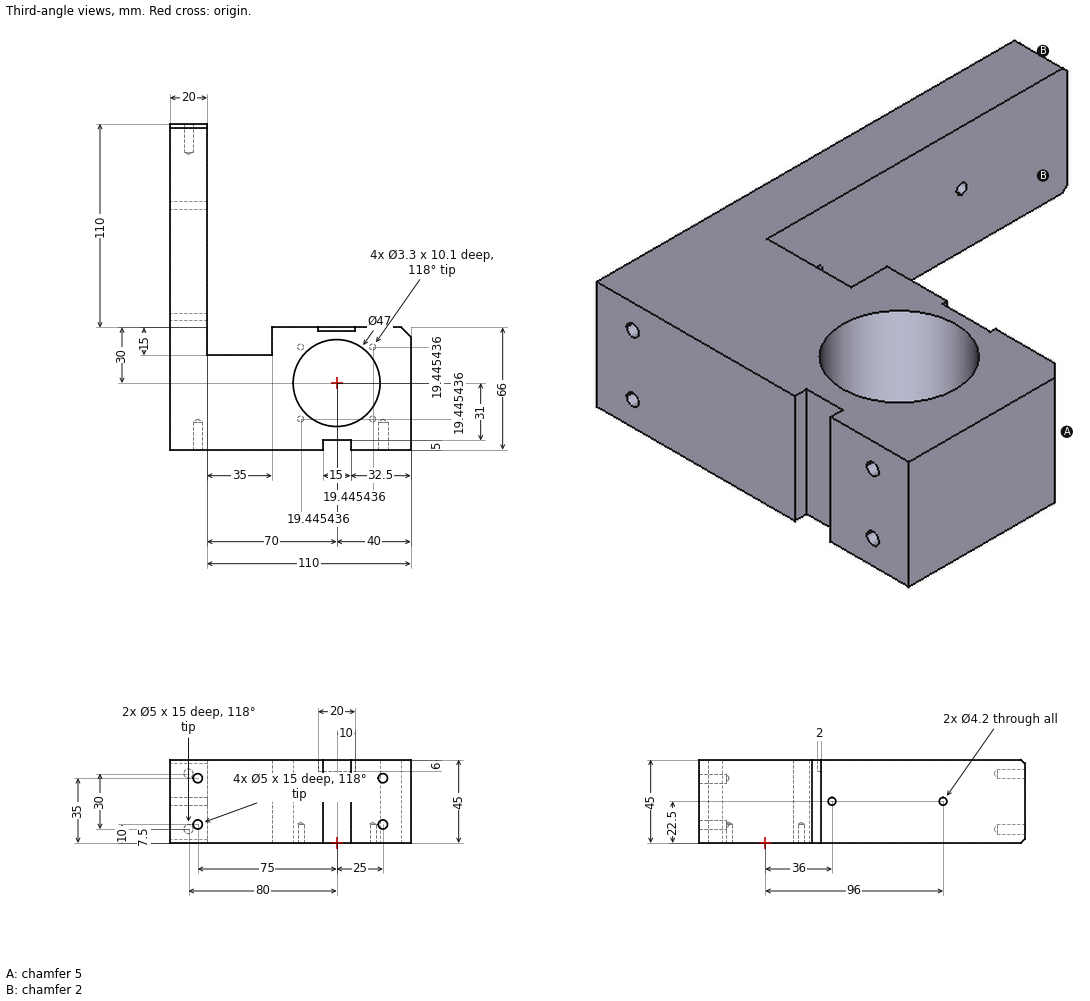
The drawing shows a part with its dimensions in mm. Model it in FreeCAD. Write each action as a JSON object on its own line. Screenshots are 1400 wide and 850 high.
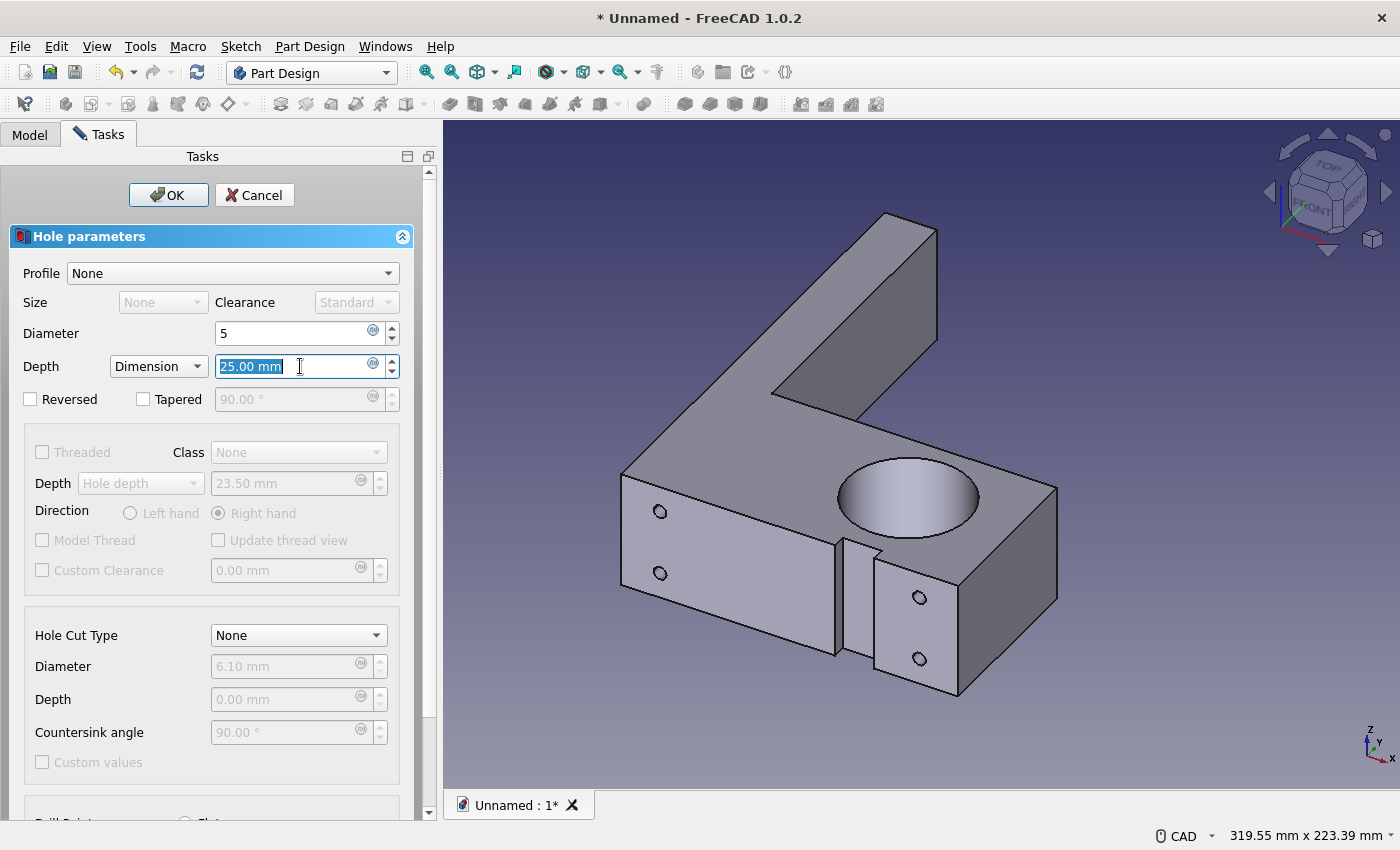
{"action": "type", "text": "15"}
{"action": "key", "text": "Tab"}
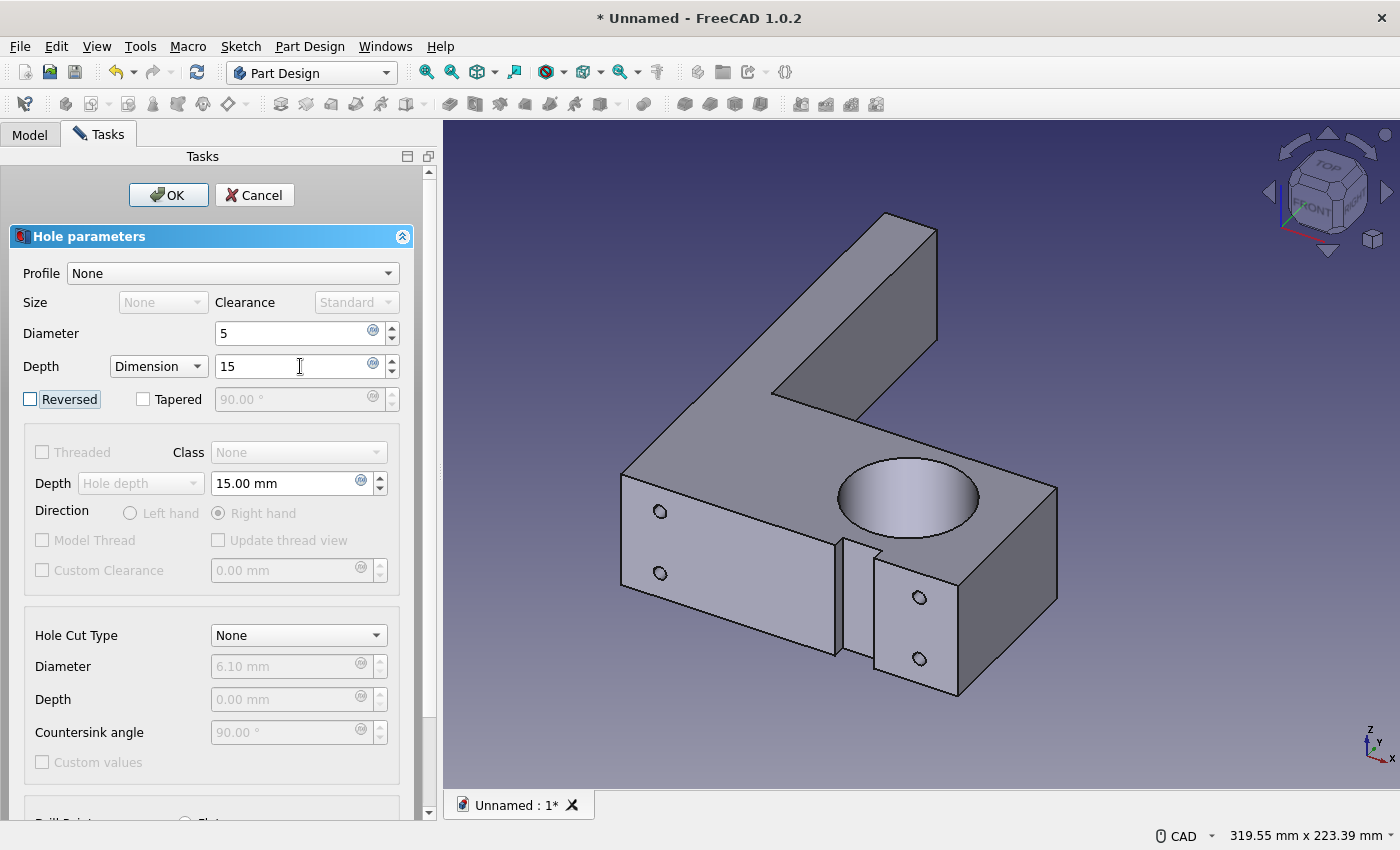
{"action": "left_click", "coordinate": [169, 195]}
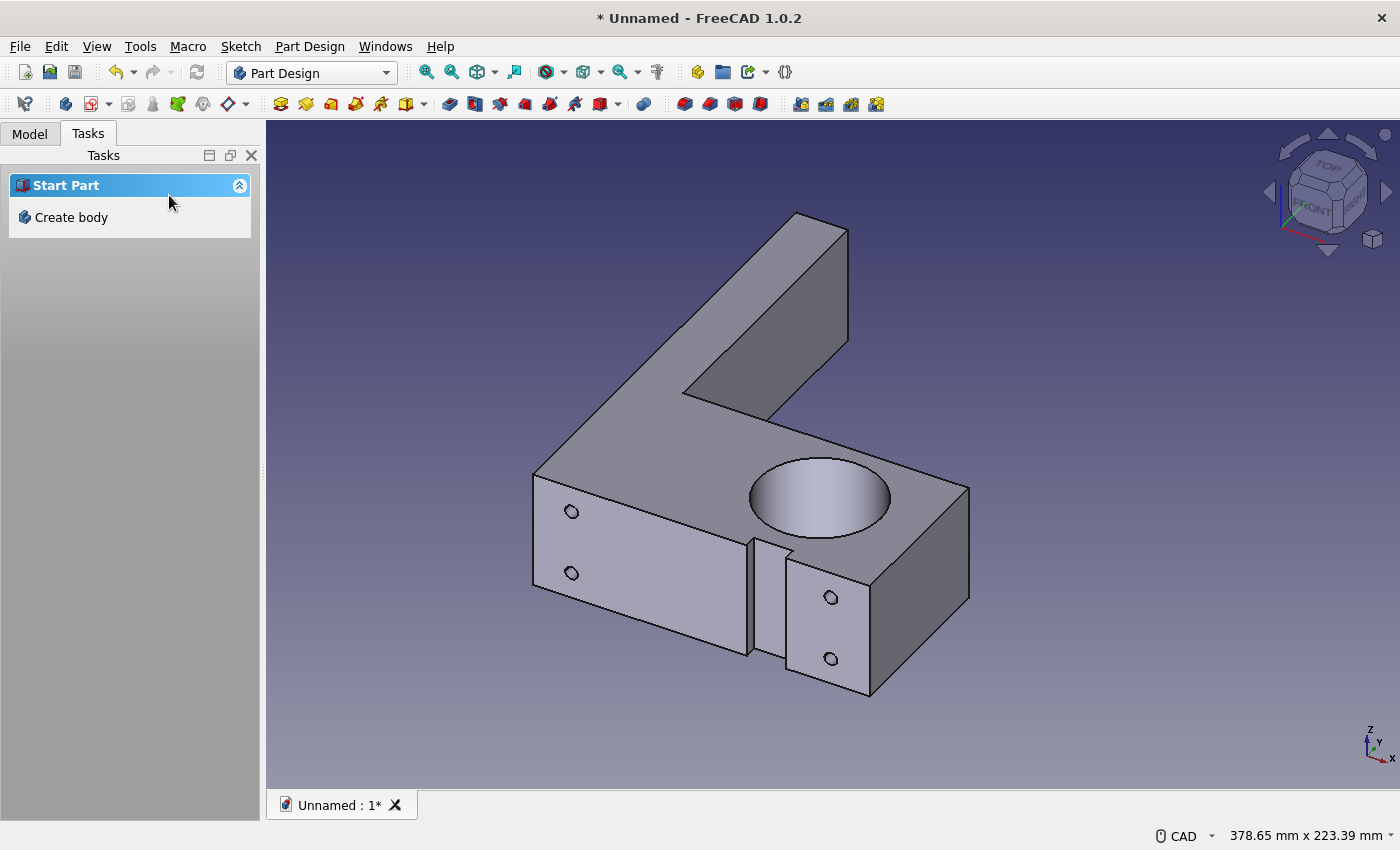
{"action": "left_click", "coordinate": [813, 319]}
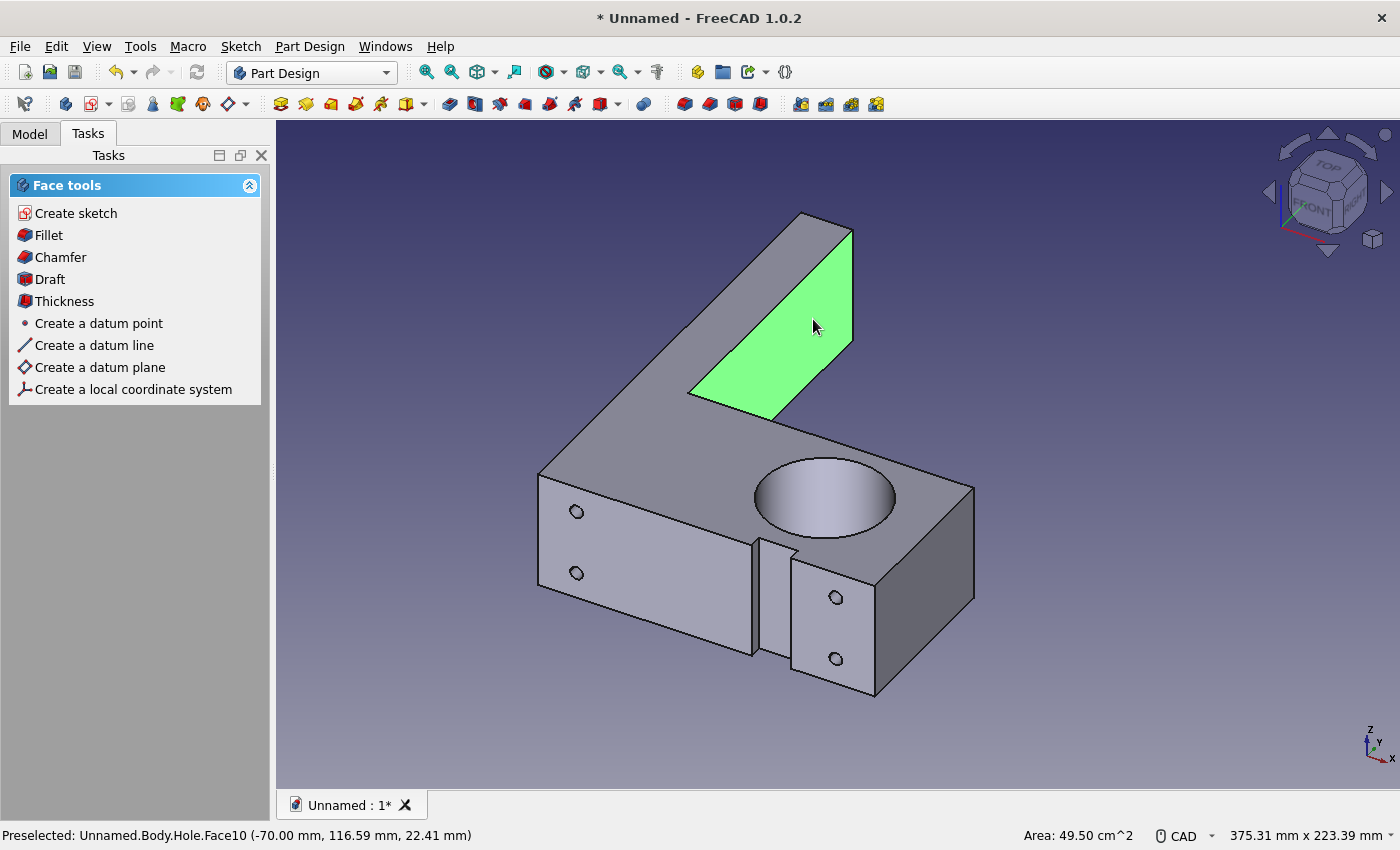
{"action": "left_click", "coordinate": [90, 104]}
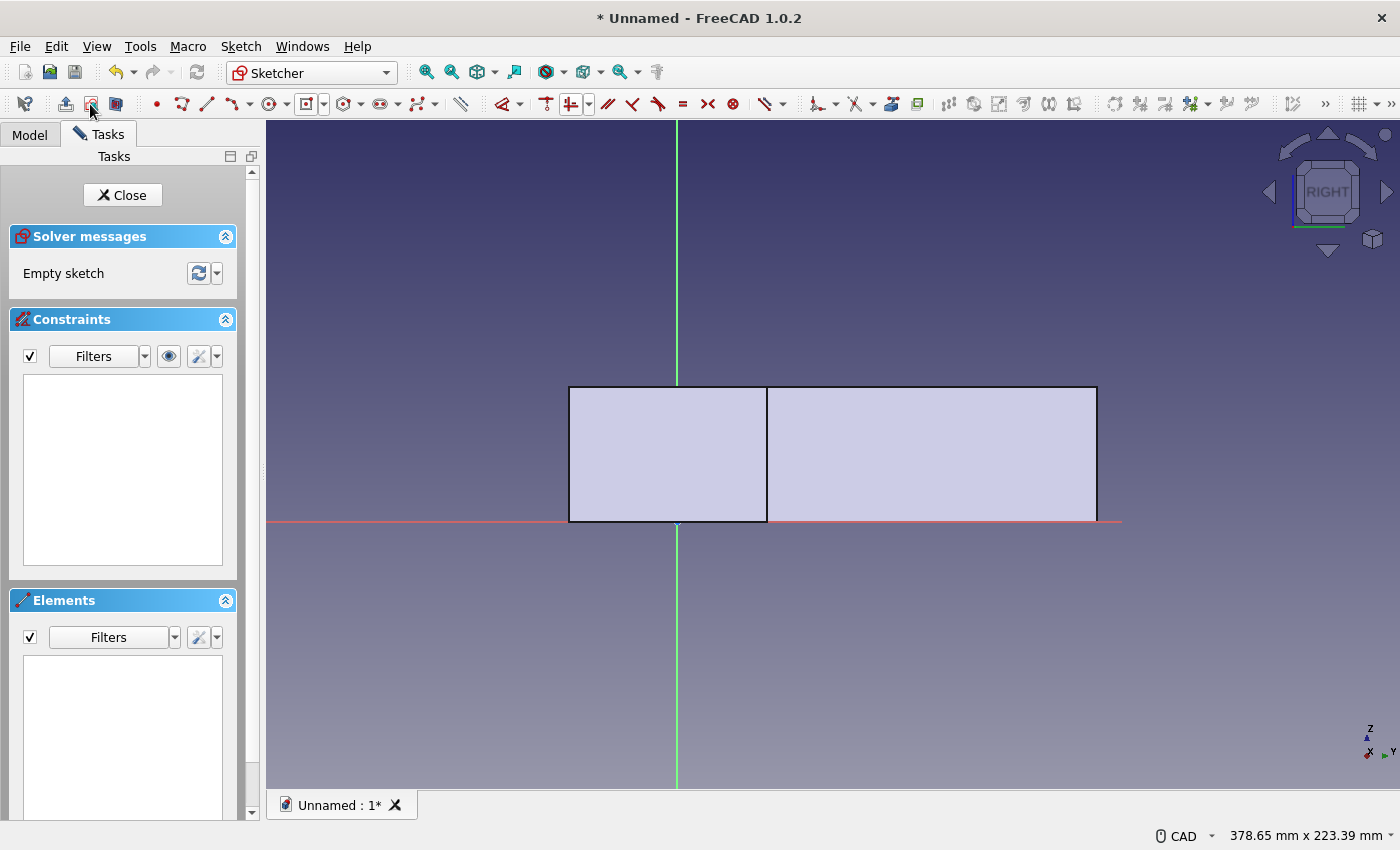
{"action": "left_click", "coordinate": [116, 104]}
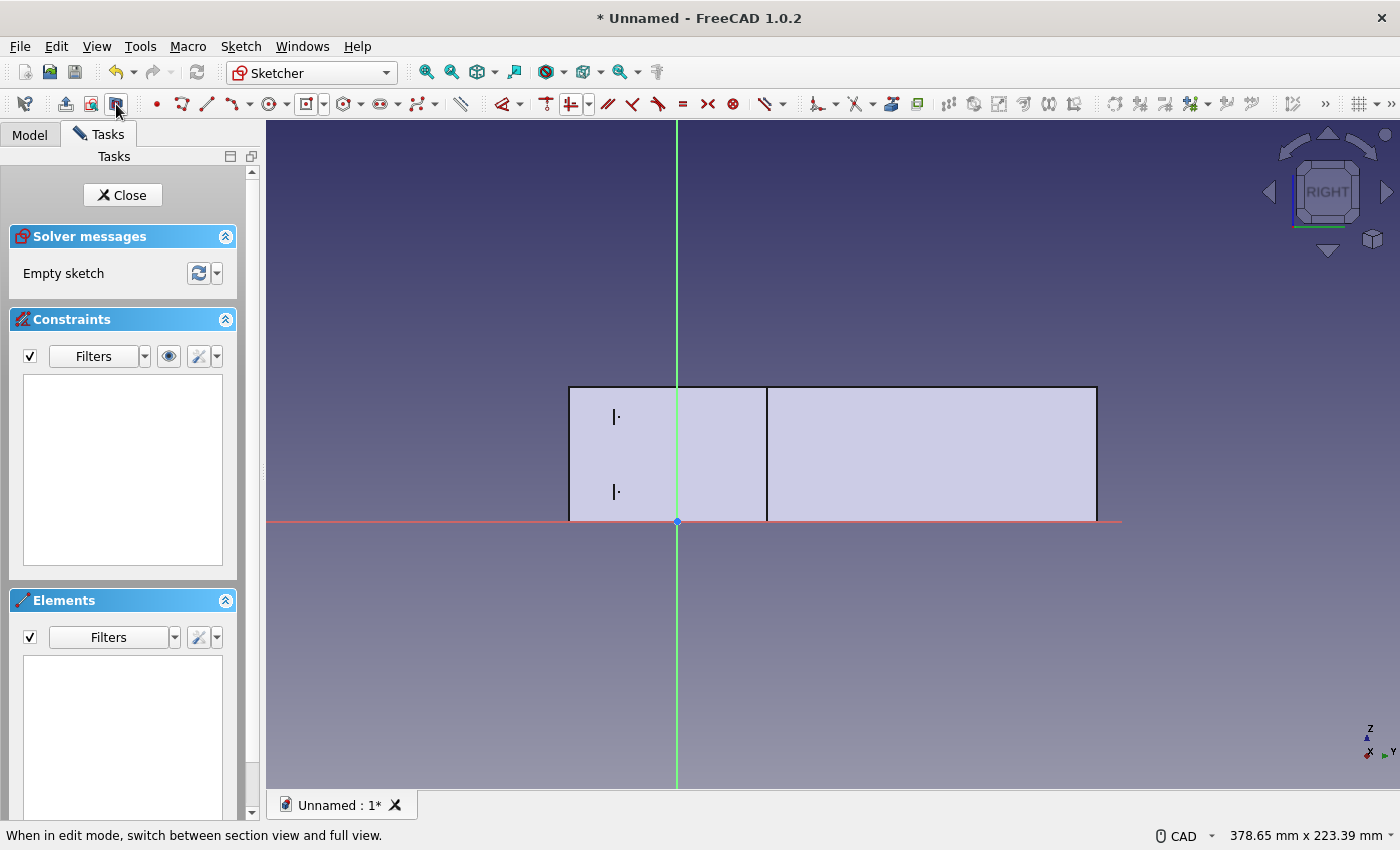
{"action": "scroll", "coordinate": [873, 510], "scroll_direction": "up", "scroll_amount": 4}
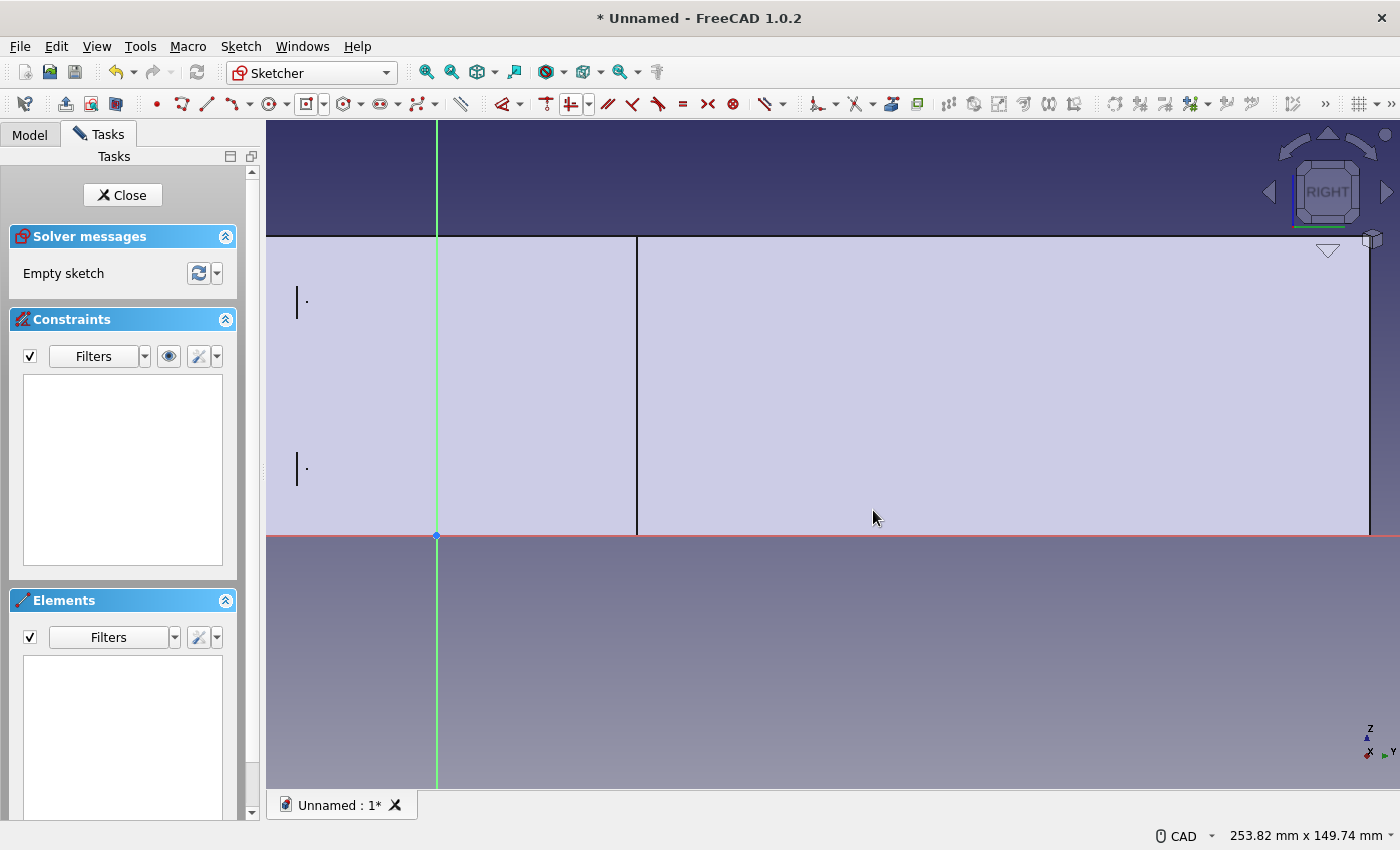
{"action": "left_click", "coordinate": [268, 104]}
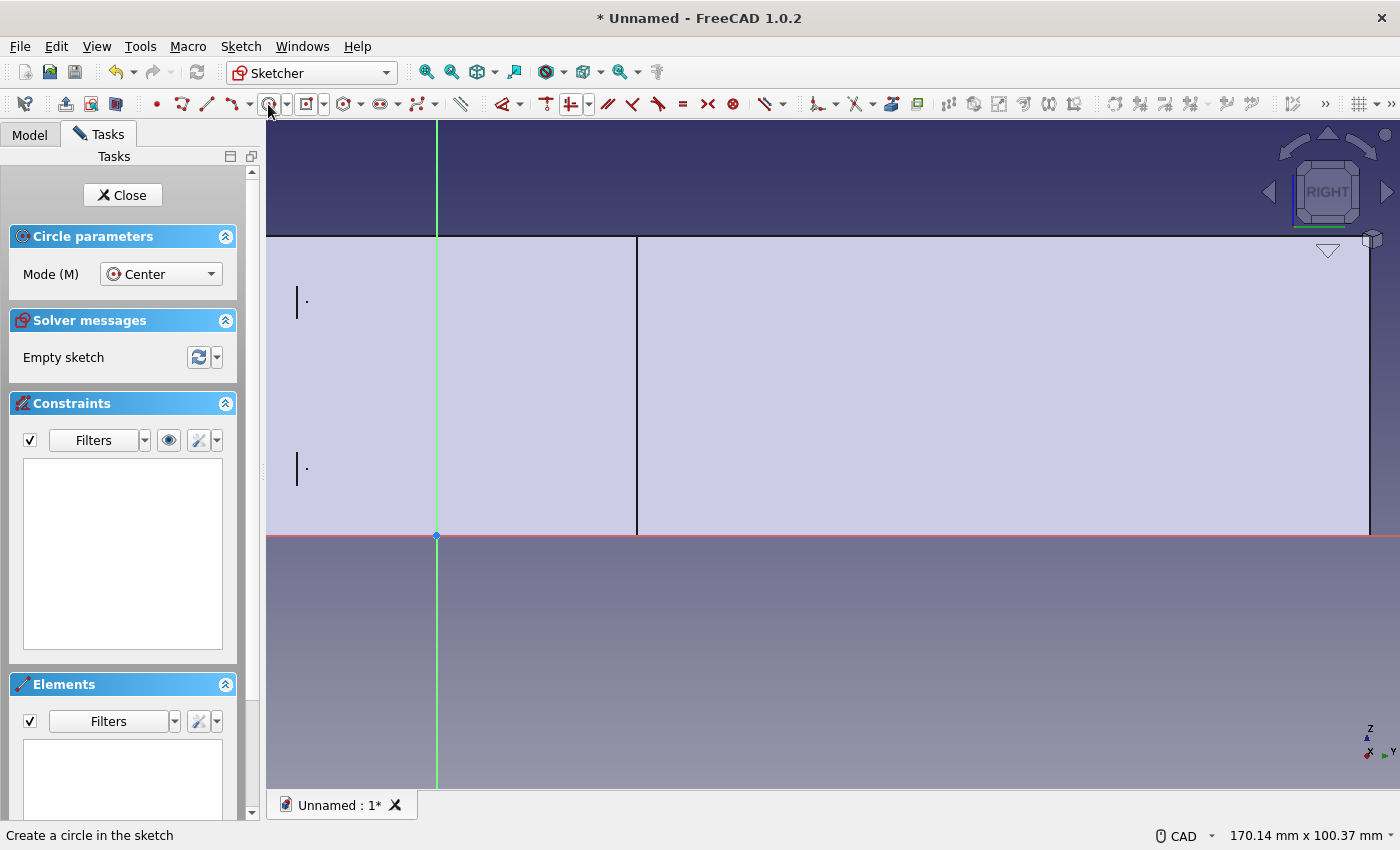
{"action": "scroll", "coordinate": [1077, 386], "scroll_direction": "up", "scroll_amount": 3}